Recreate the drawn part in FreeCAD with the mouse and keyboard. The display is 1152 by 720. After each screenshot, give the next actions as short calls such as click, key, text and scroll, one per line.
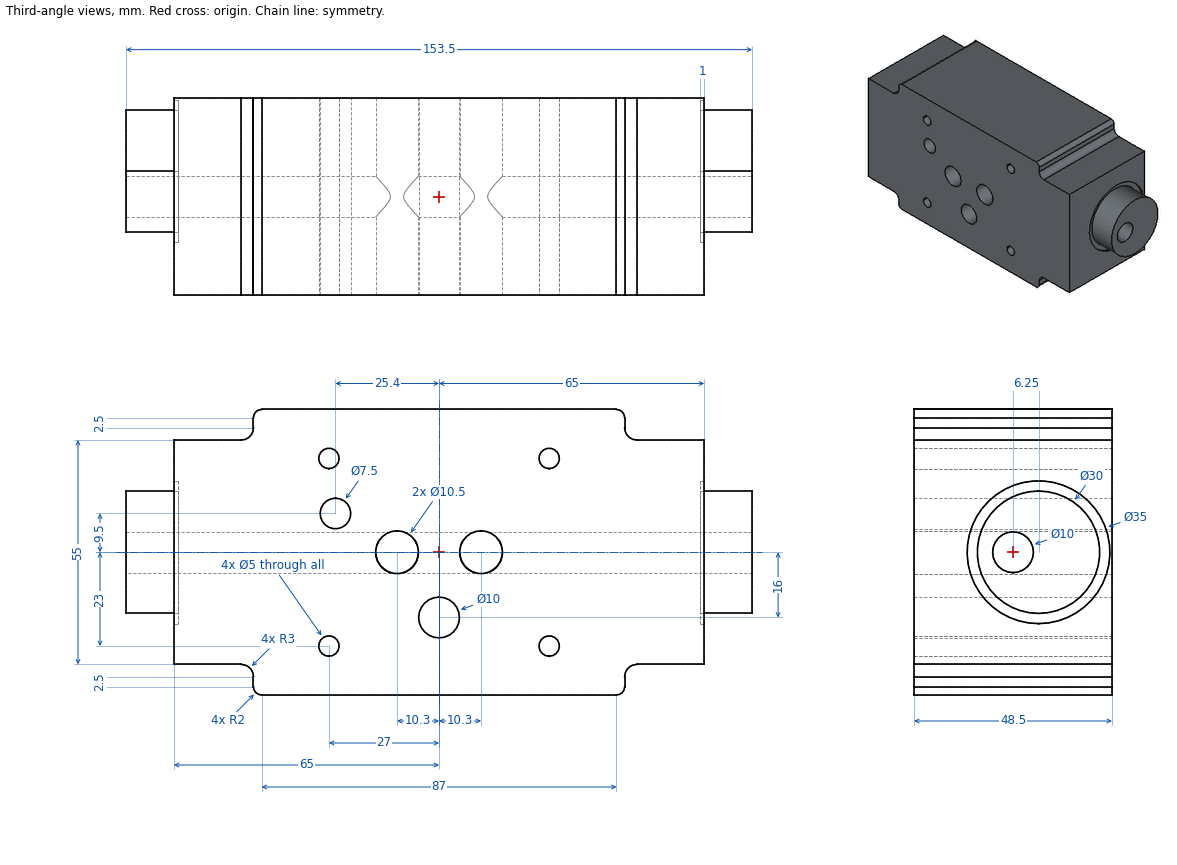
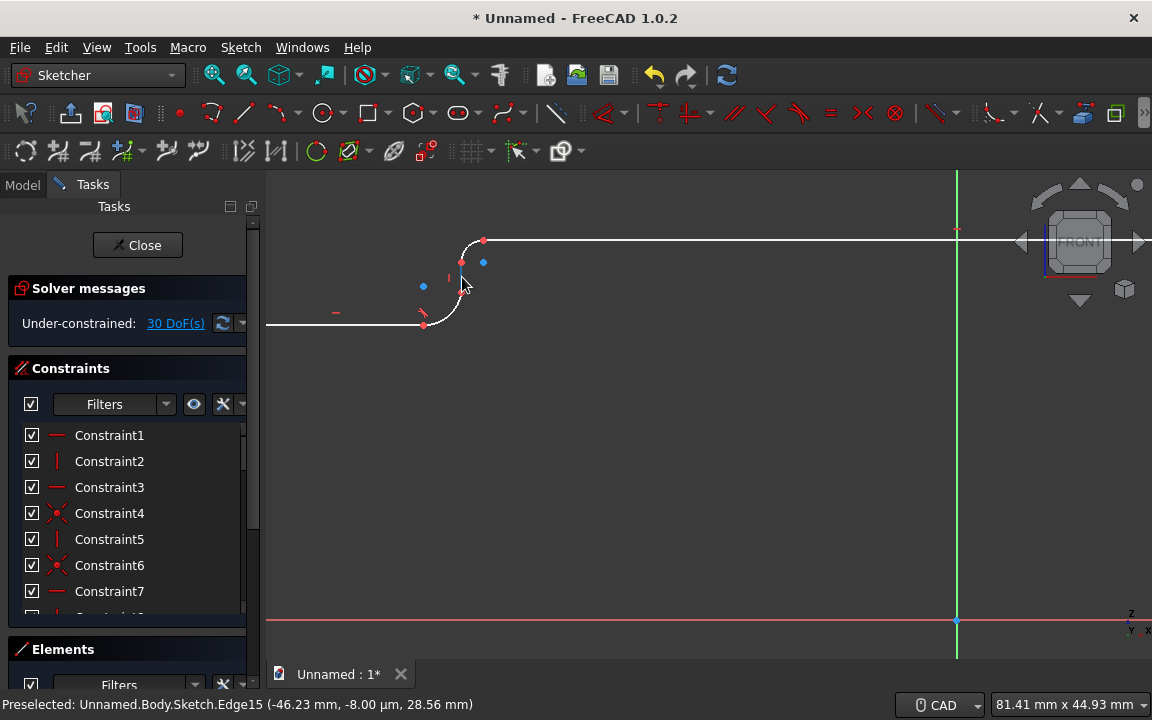
click(461, 278)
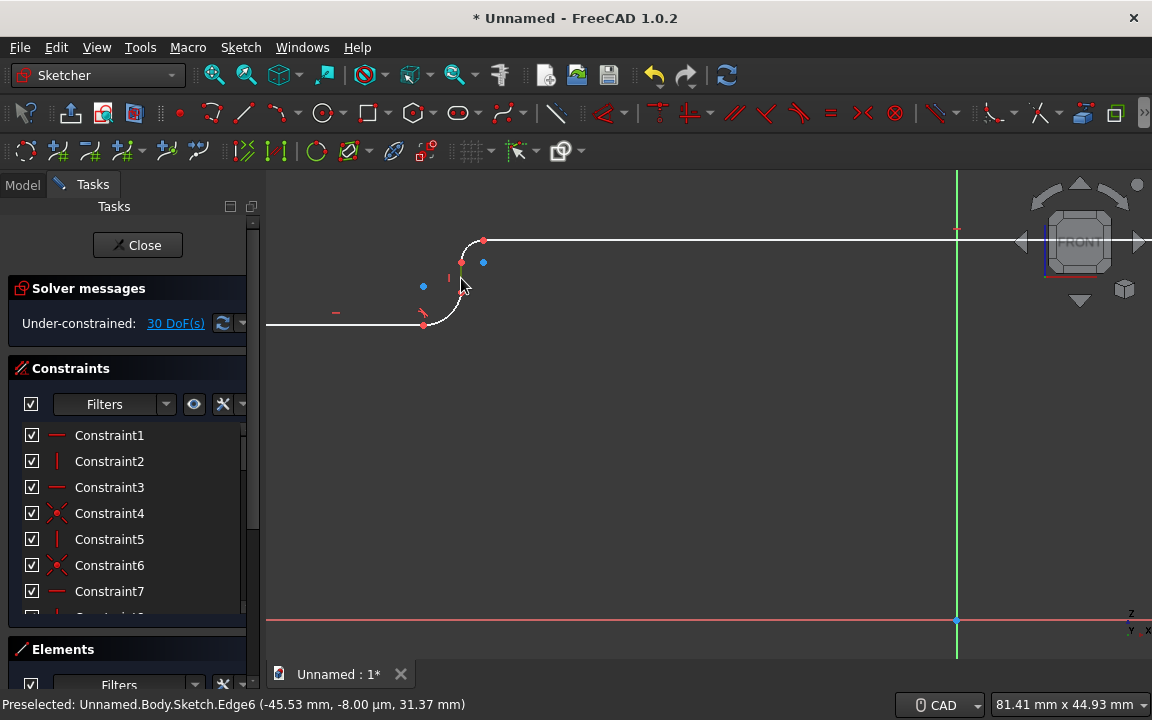
click(439, 322)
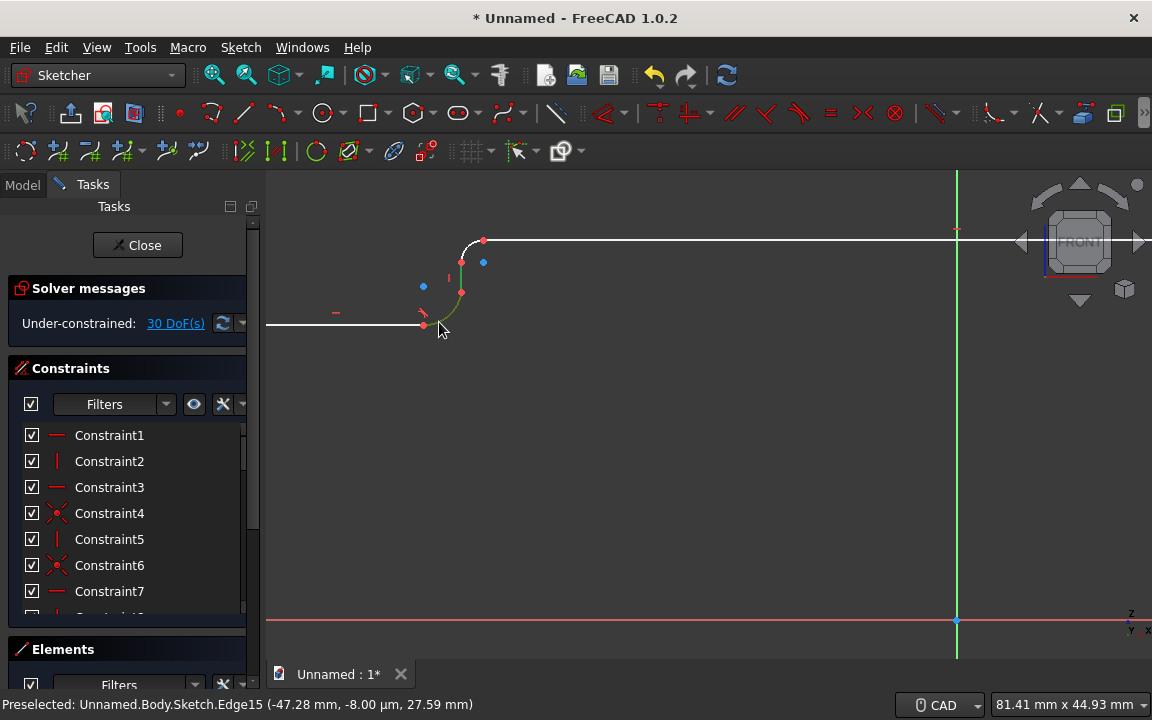
click(800, 114)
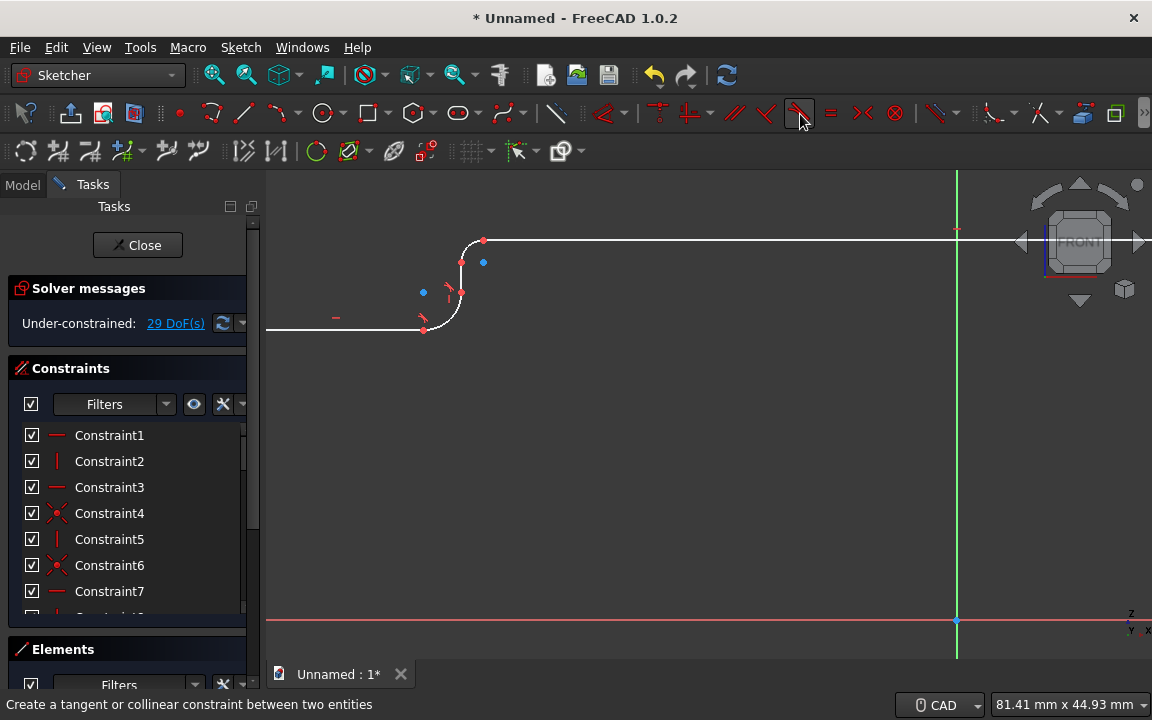
click(461, 280)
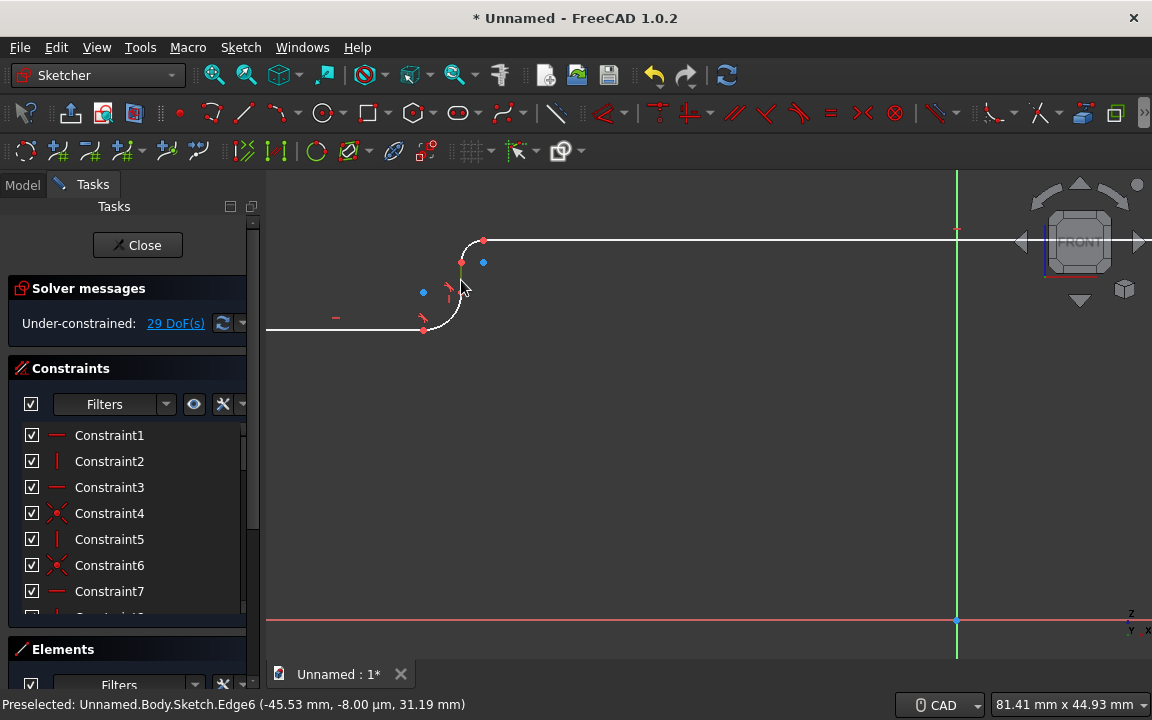
scroll(473, 243, up, 2)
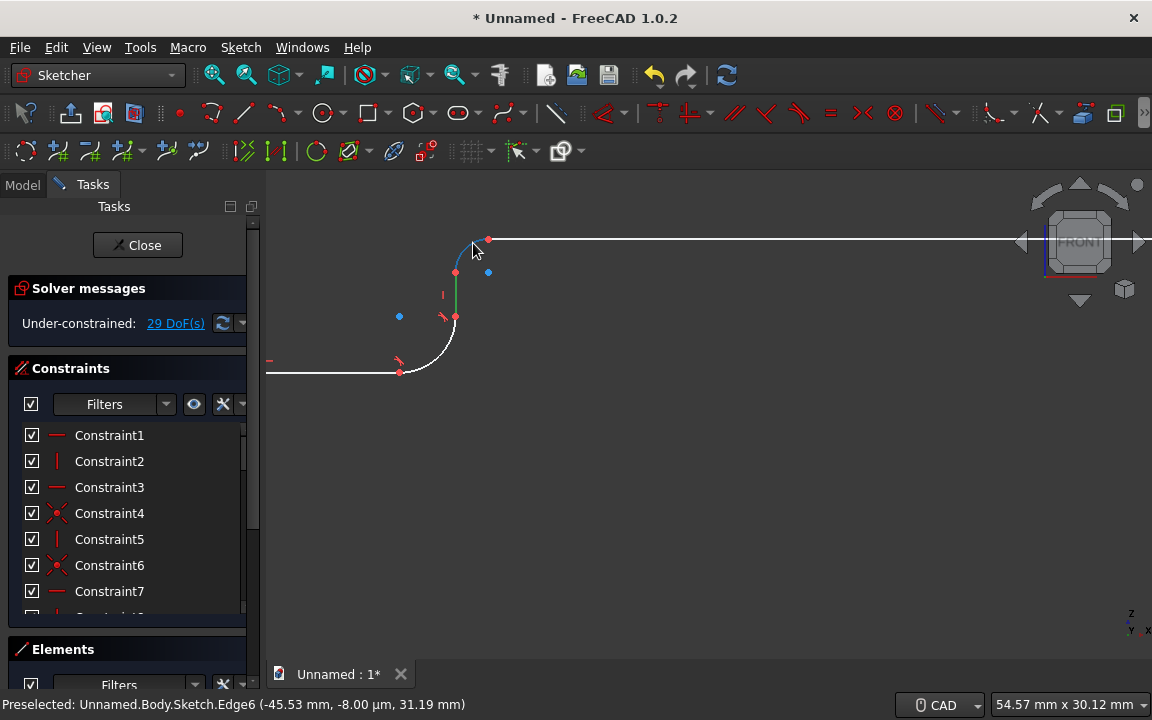
click(474, 243)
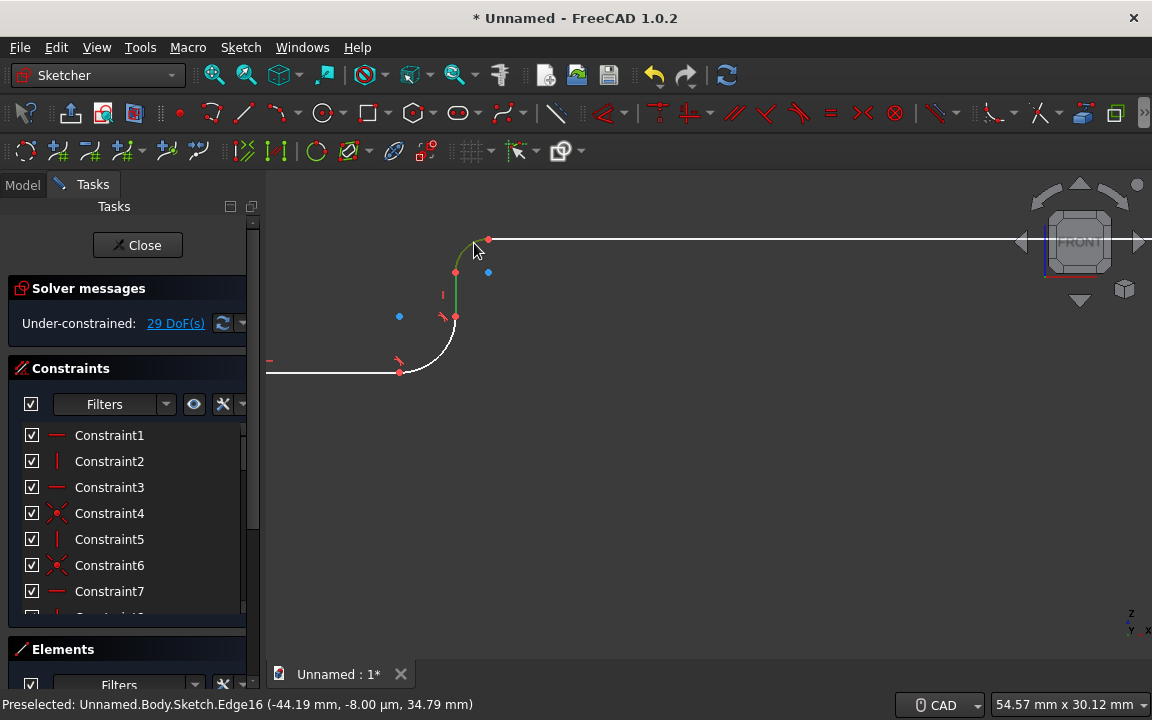
click(800, 114)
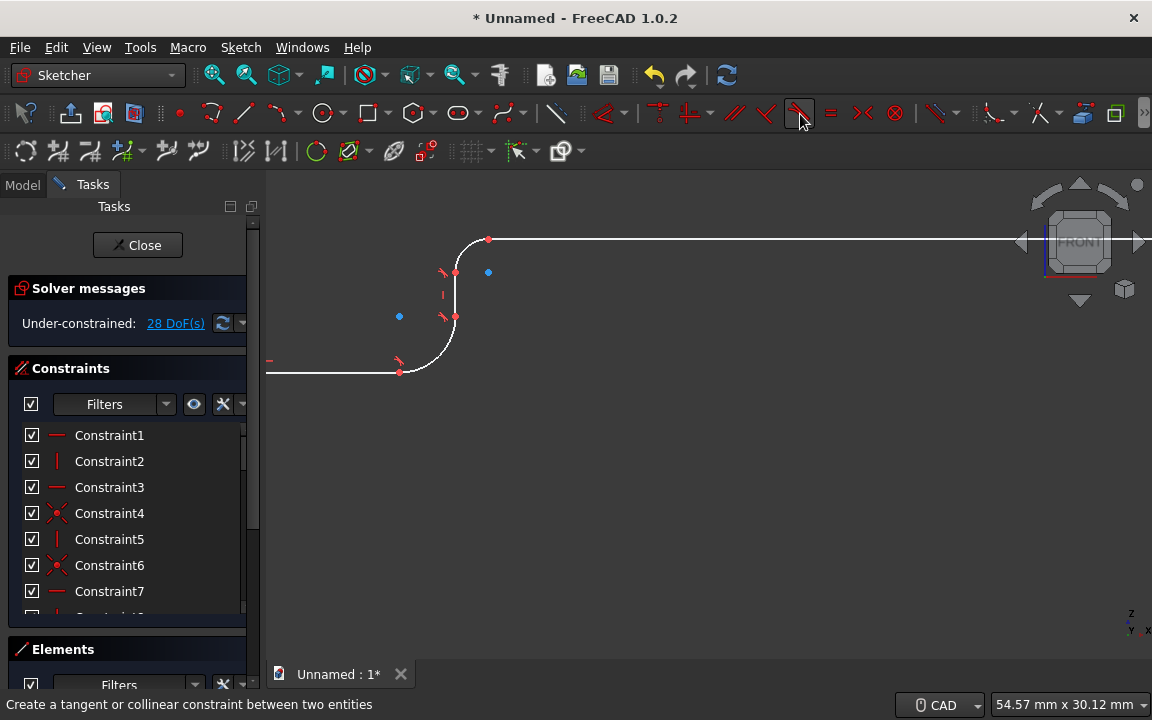
scroll(459, 286, down, 7)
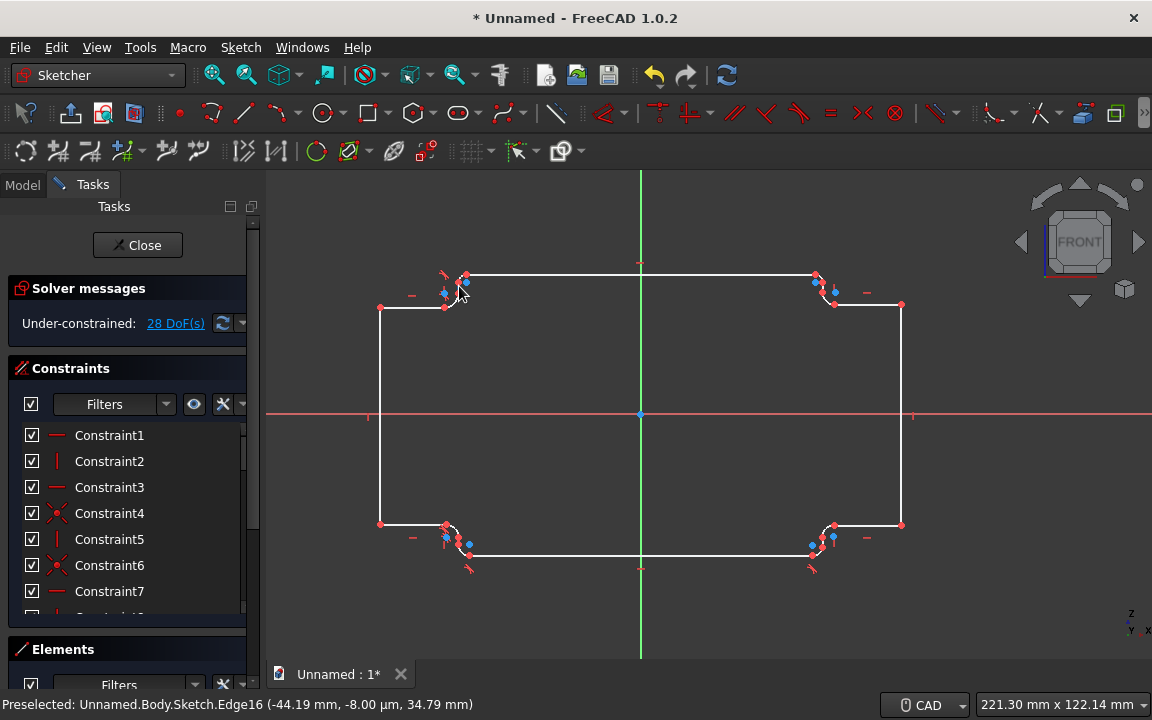
click(571, 275)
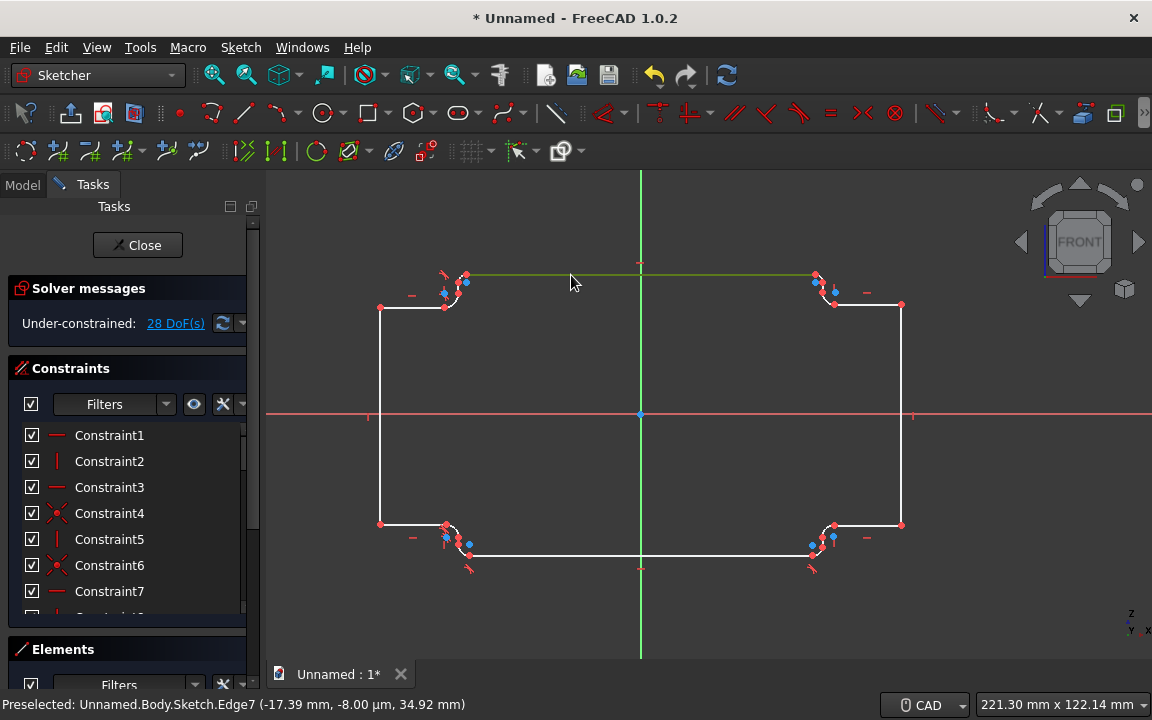
scroll(461, 277, up, 4)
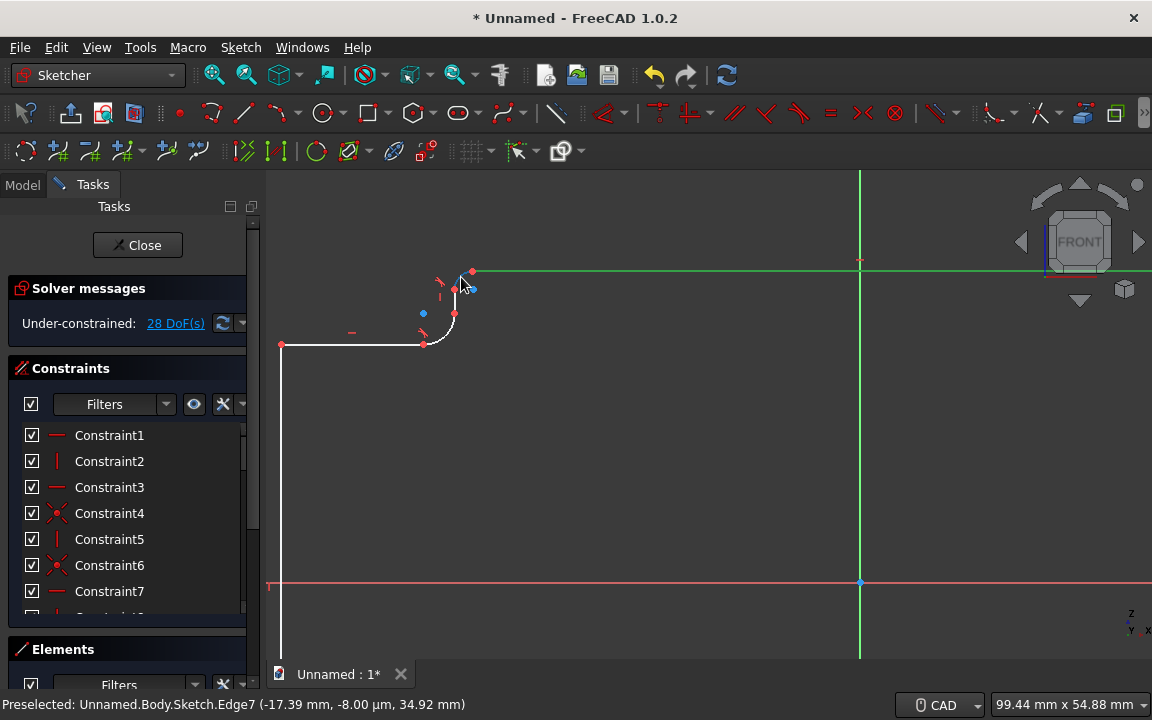
click(460, 277)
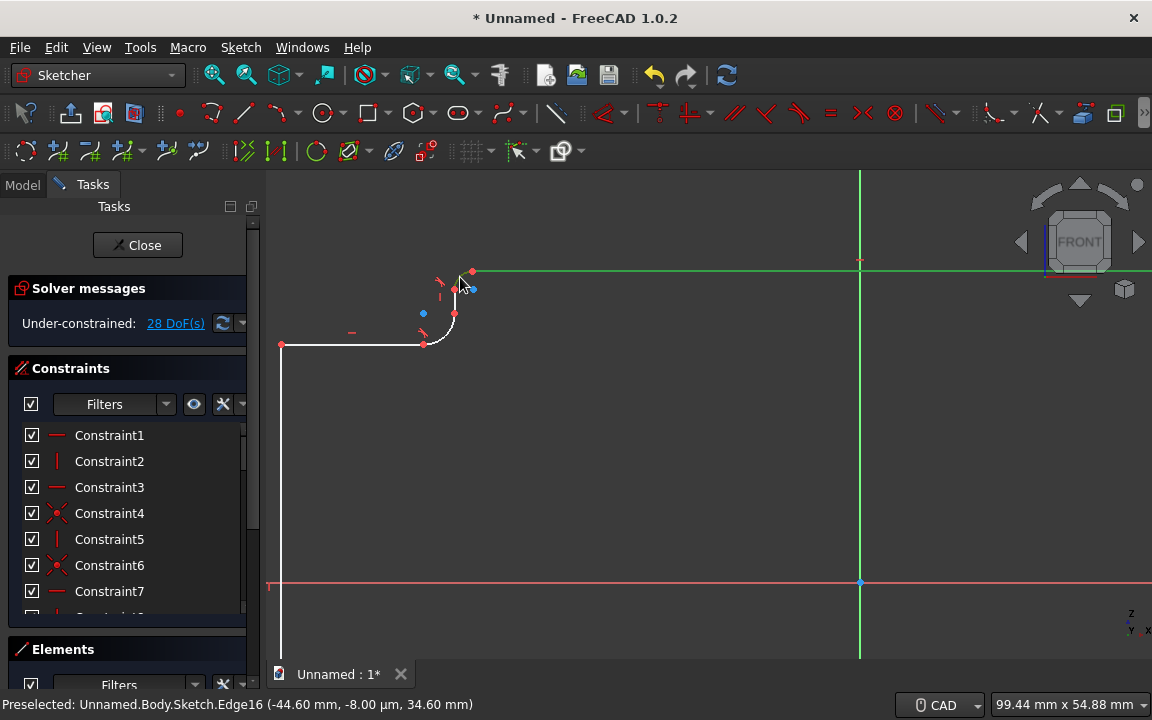
click(800, 114)